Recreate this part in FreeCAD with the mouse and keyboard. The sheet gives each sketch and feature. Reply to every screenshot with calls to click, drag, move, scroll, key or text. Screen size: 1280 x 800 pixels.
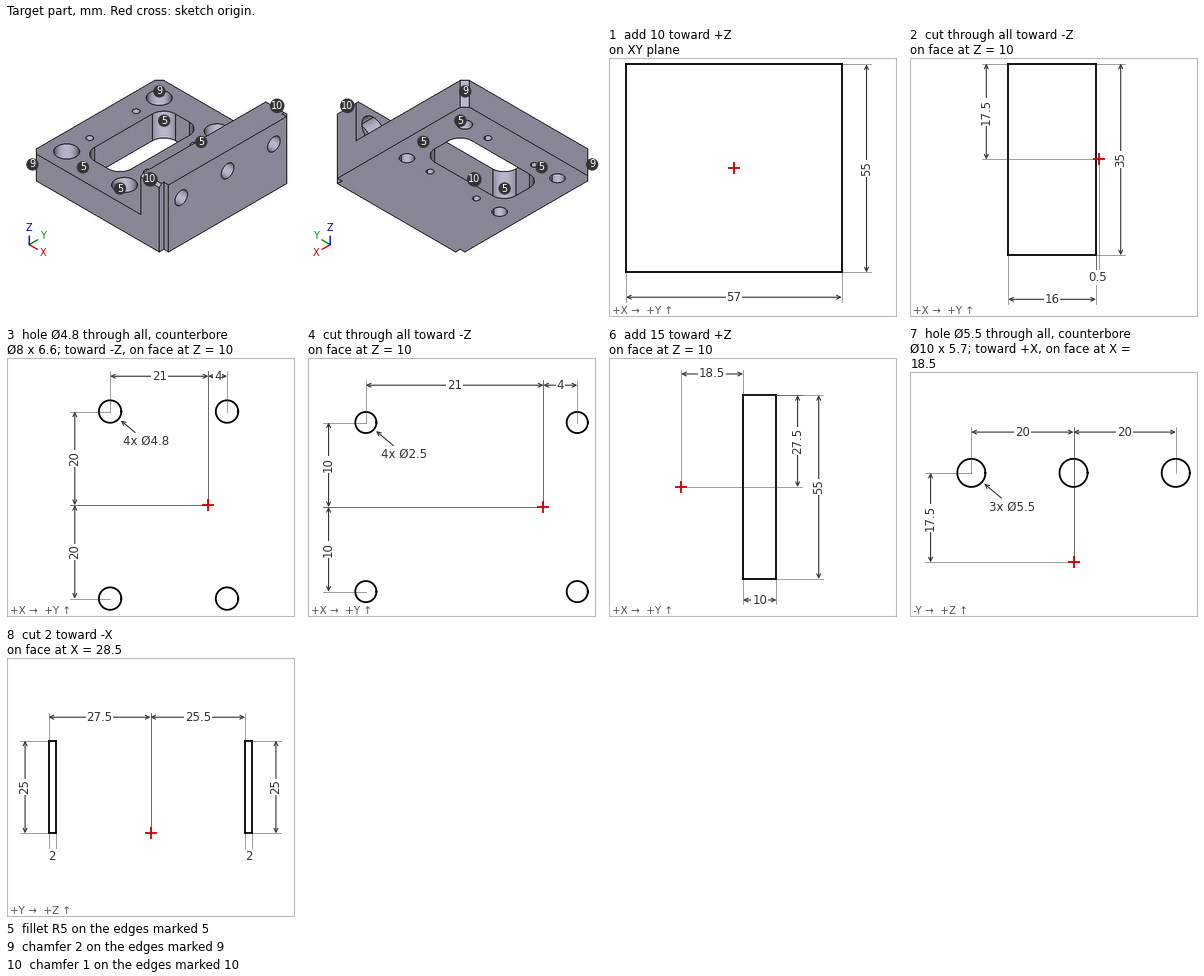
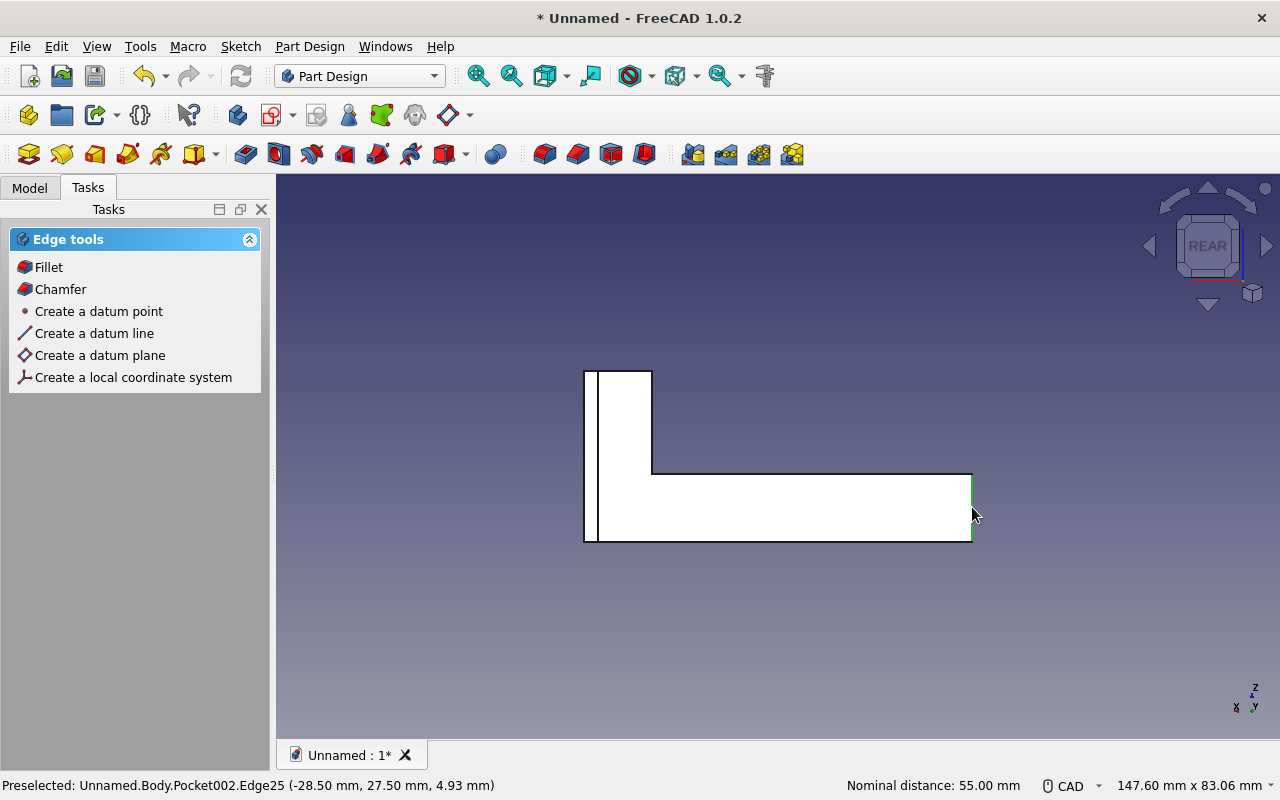
click(578, 154)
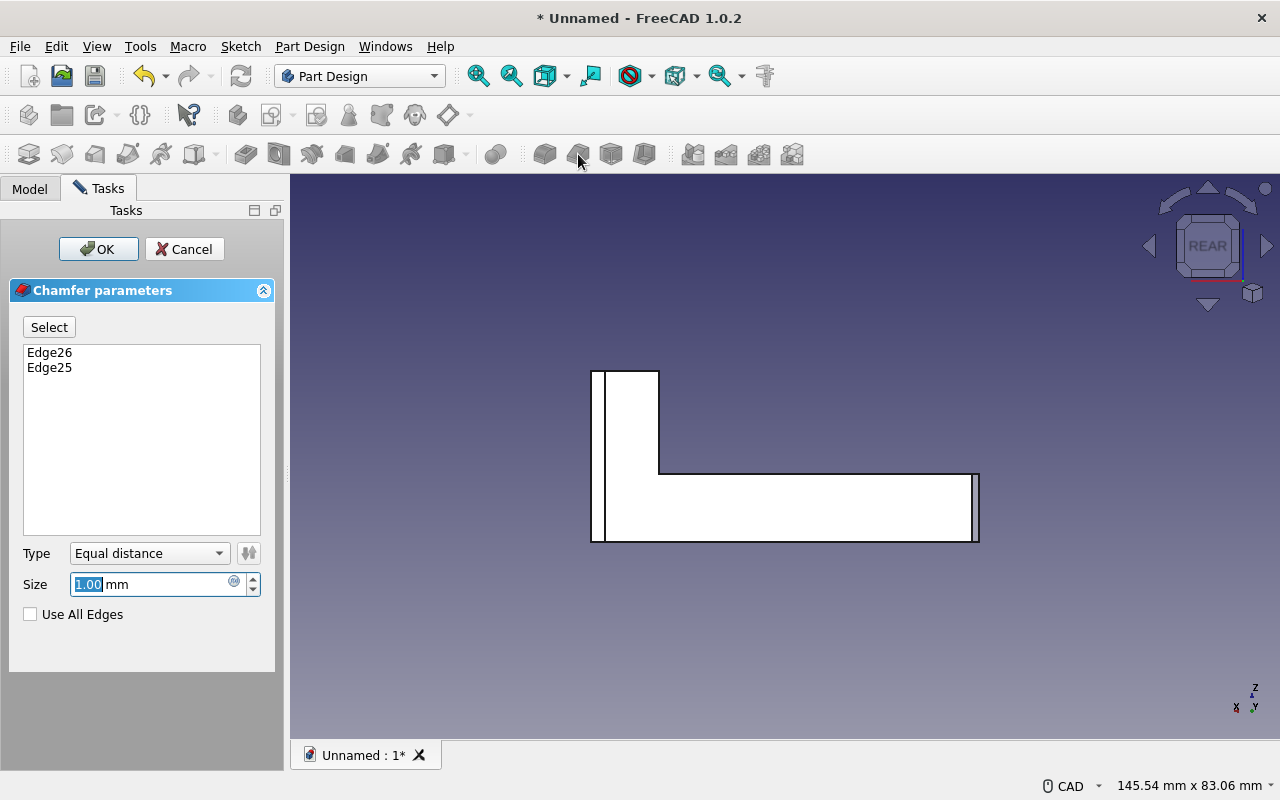
text(2)
key(Tab)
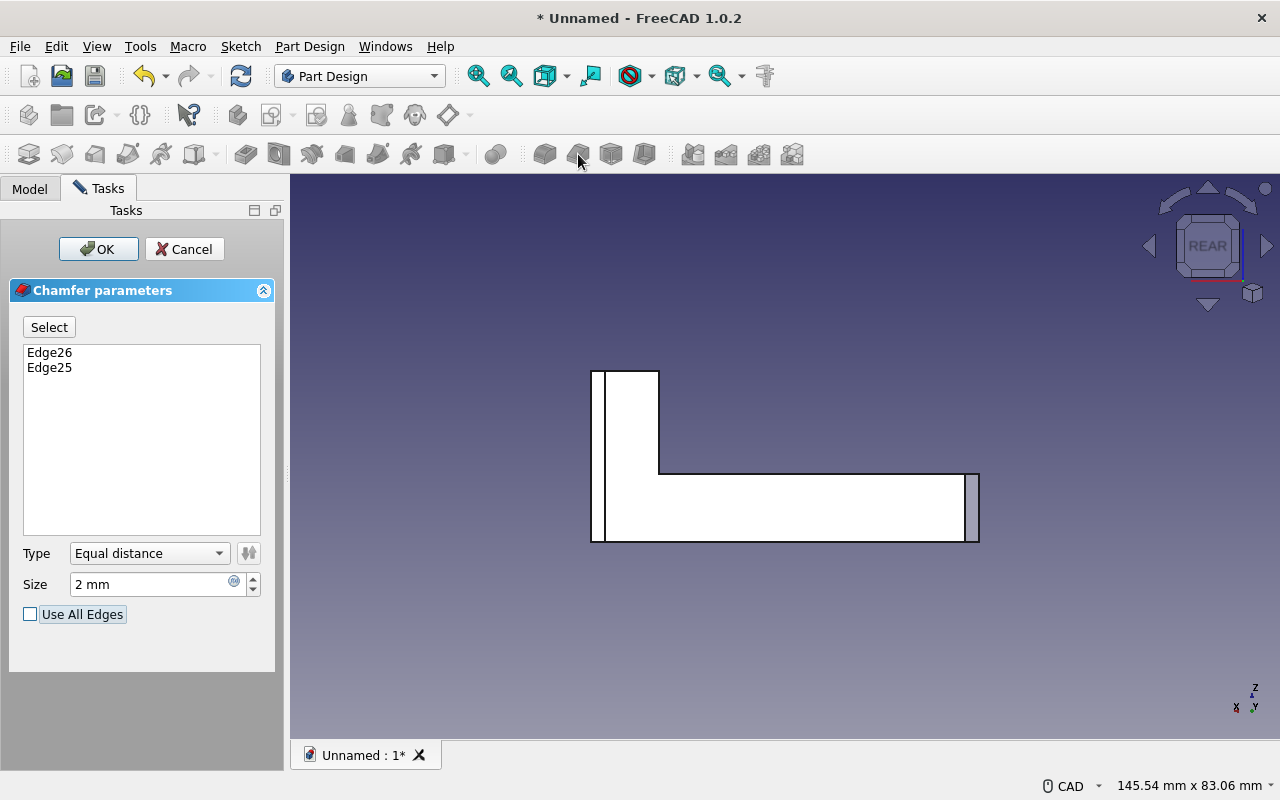
click(99, 249)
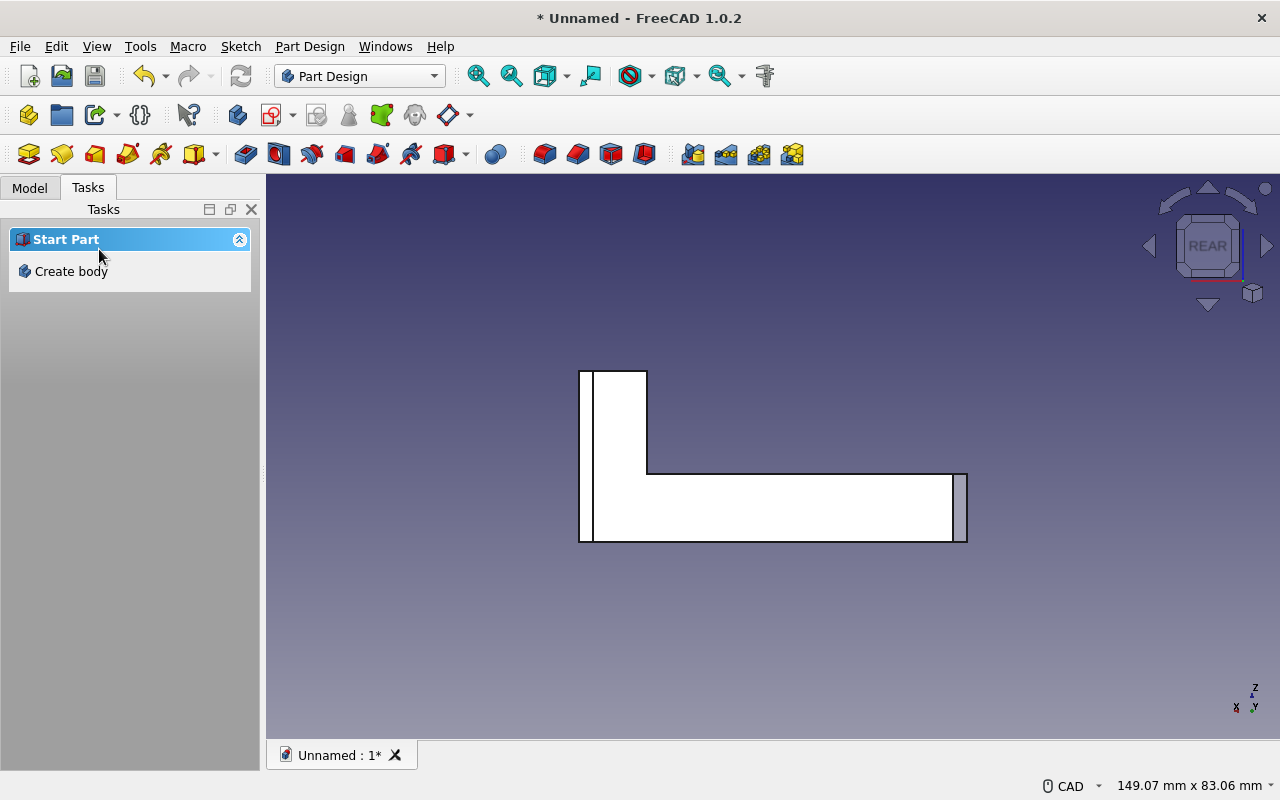
key(v)
key(f)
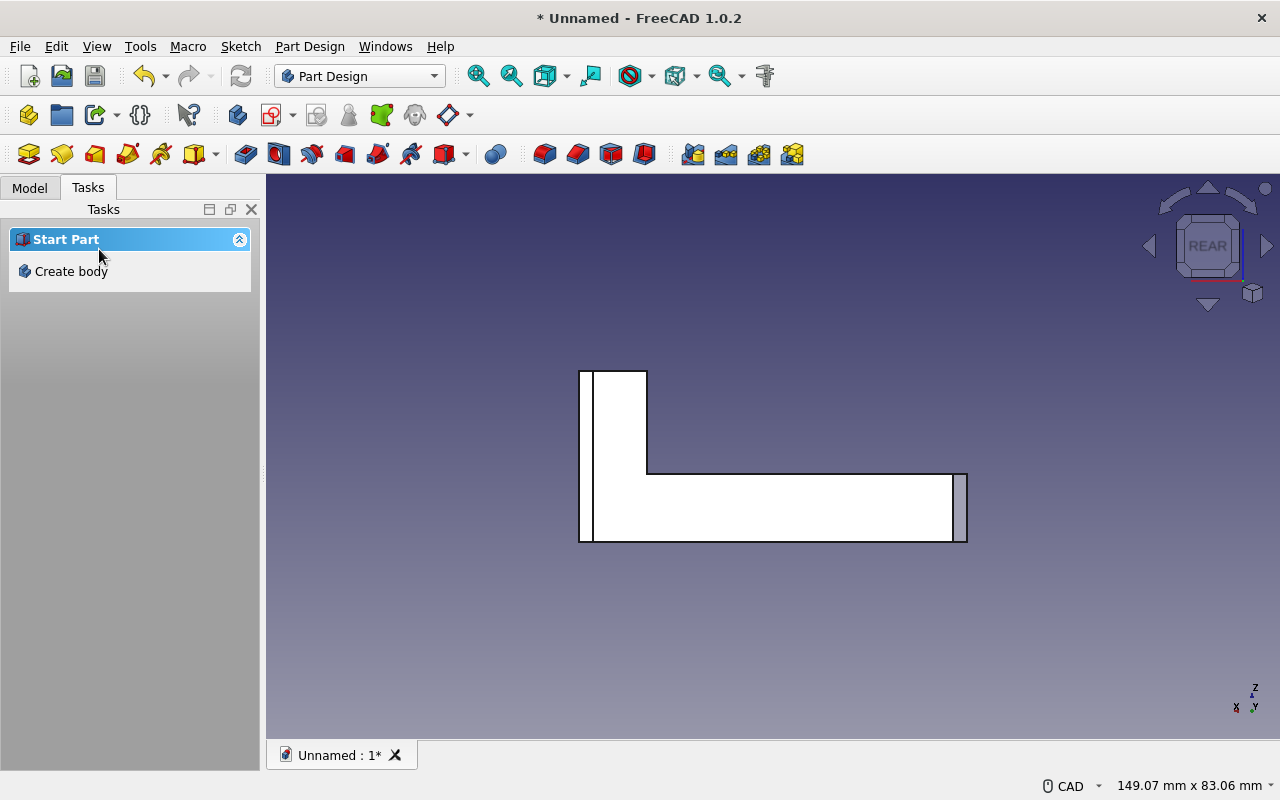
click(620, 370)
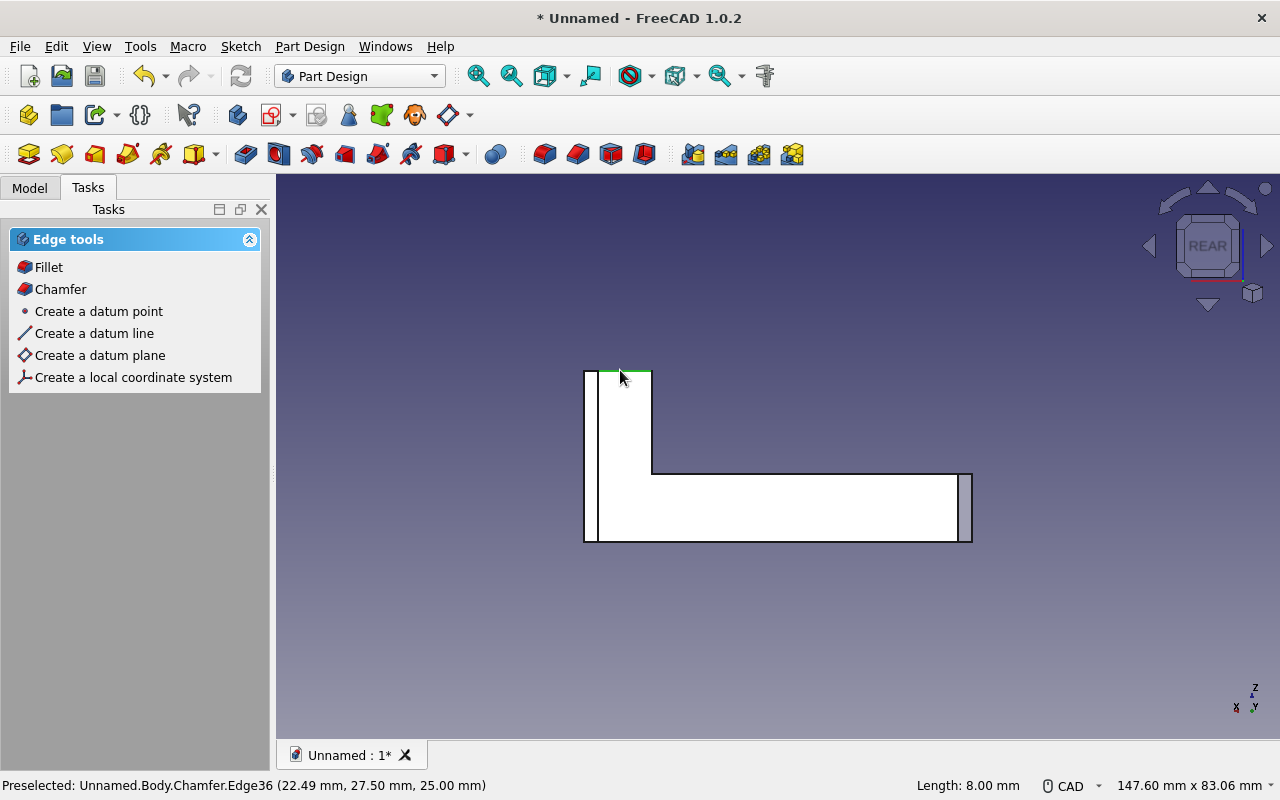
key(0)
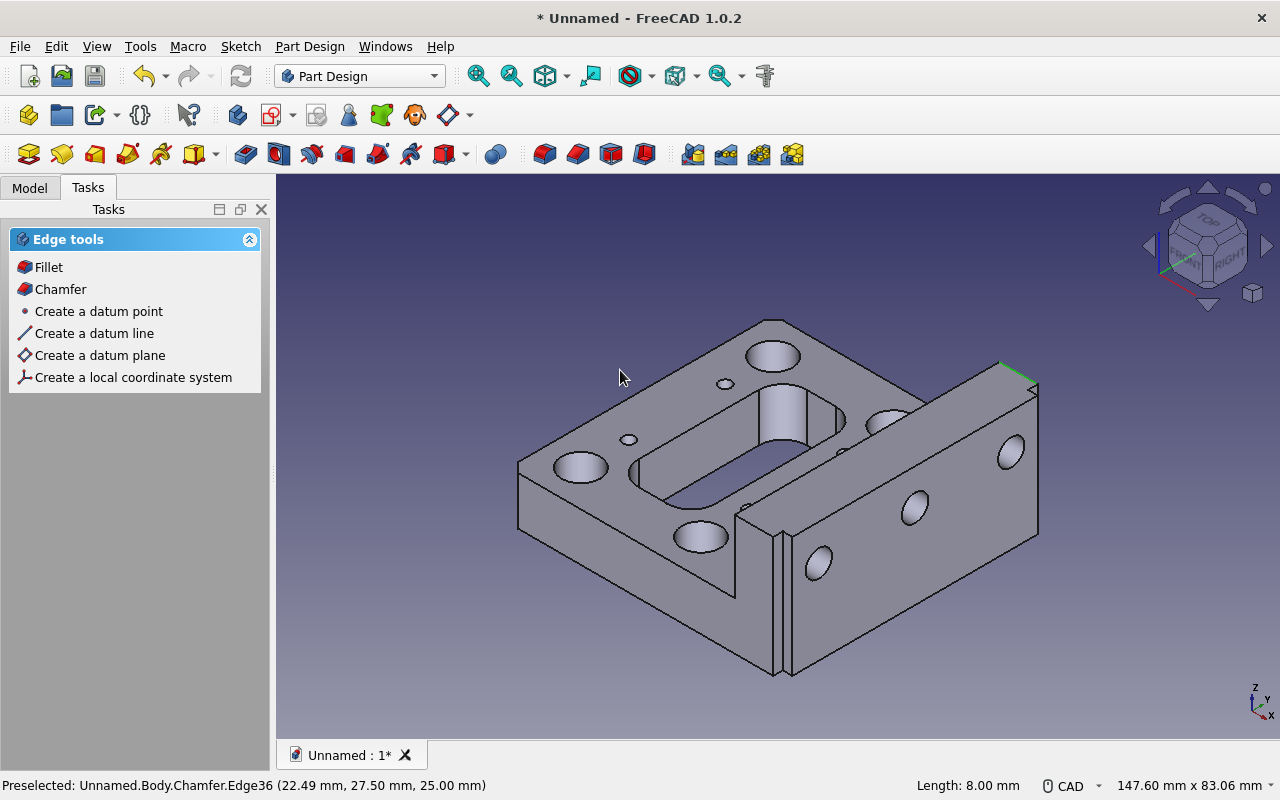
click(754, 525, ctrl)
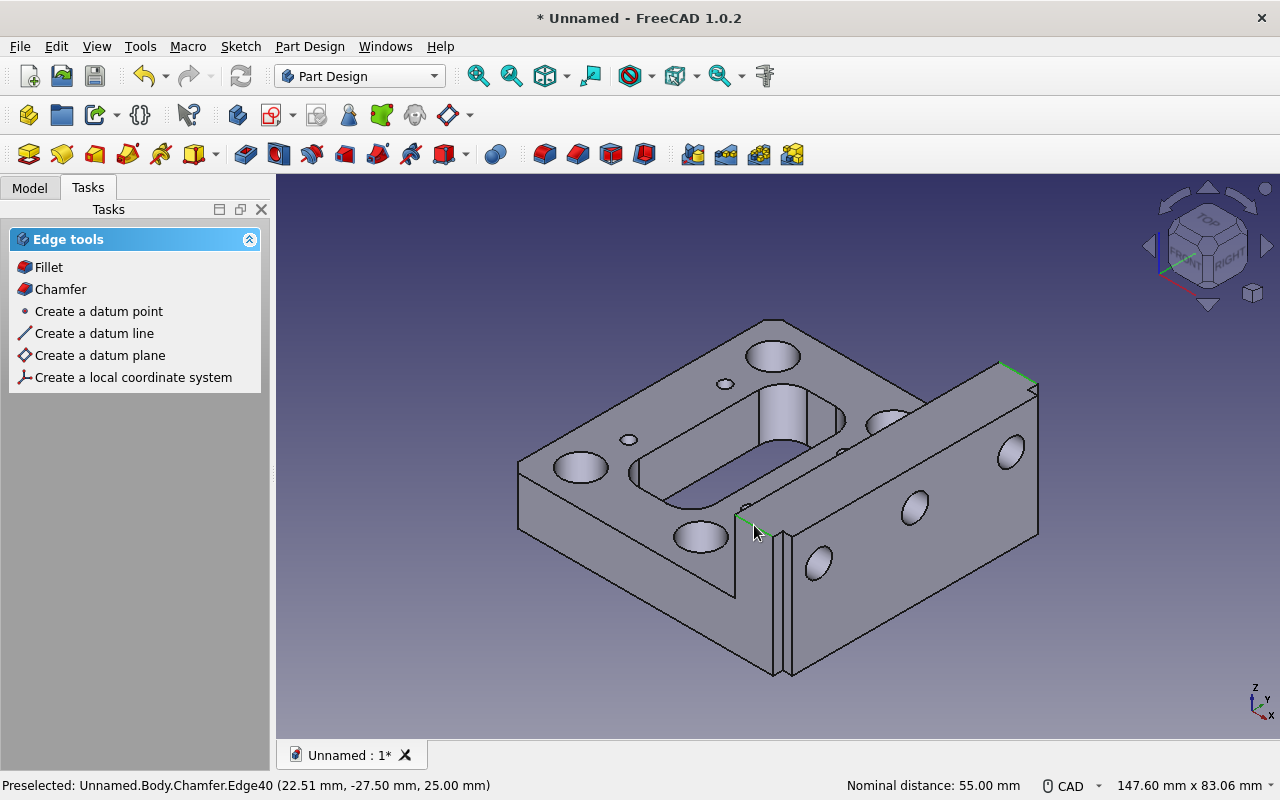
click(578, 154)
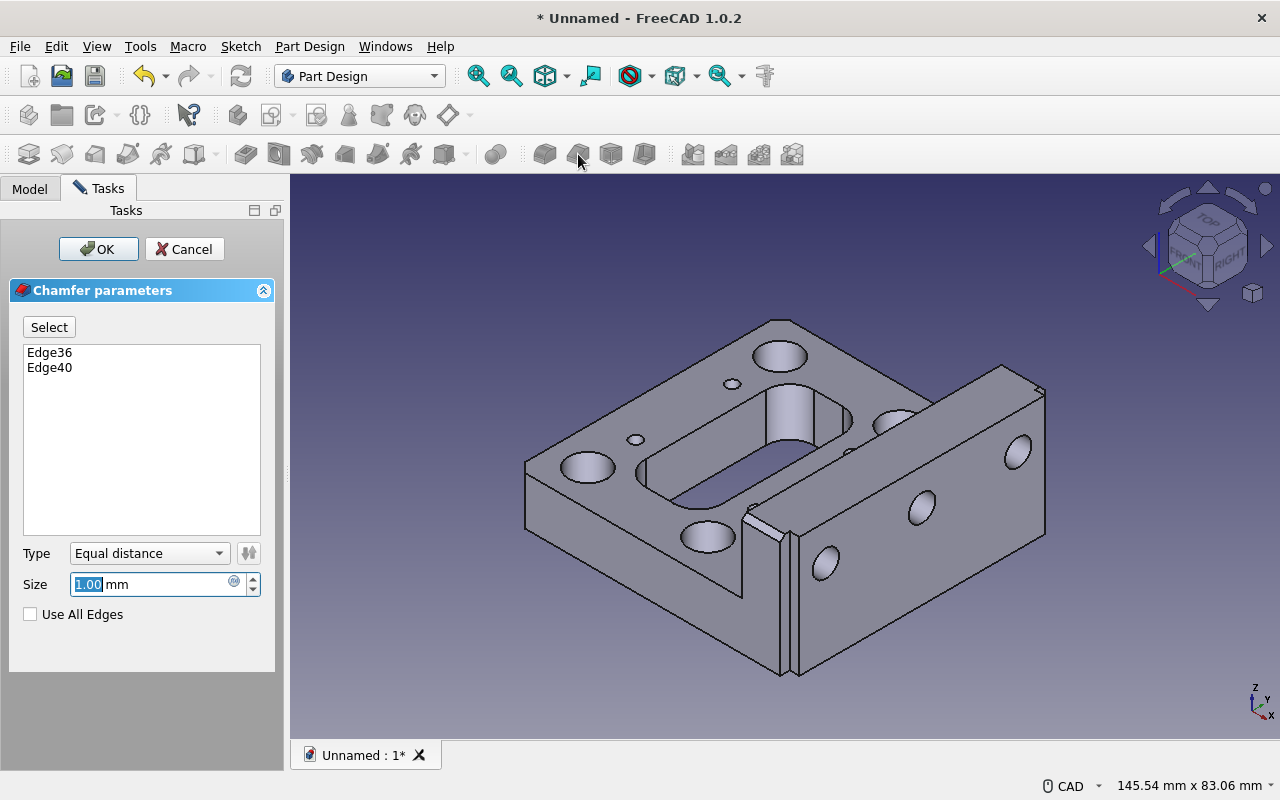
text(1)
key(Tab)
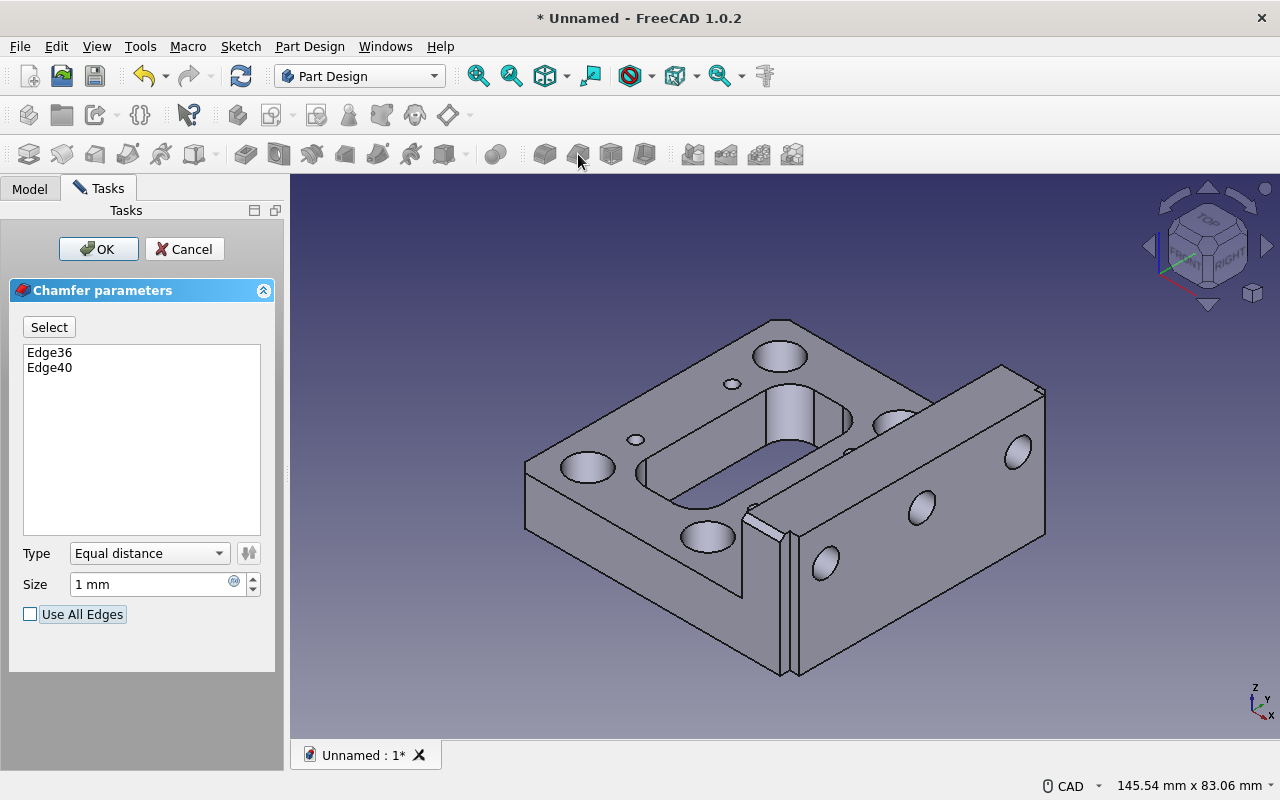
click(99, 249)